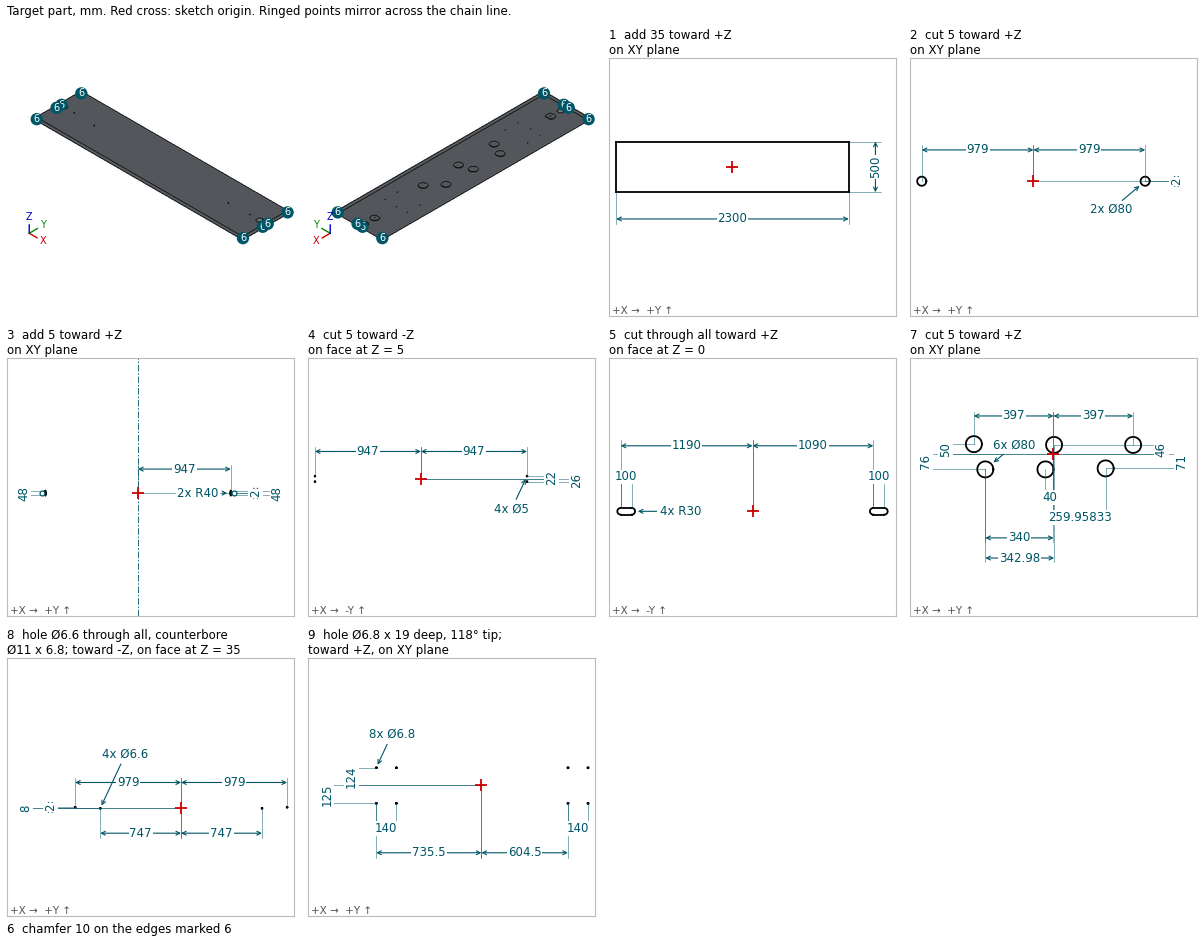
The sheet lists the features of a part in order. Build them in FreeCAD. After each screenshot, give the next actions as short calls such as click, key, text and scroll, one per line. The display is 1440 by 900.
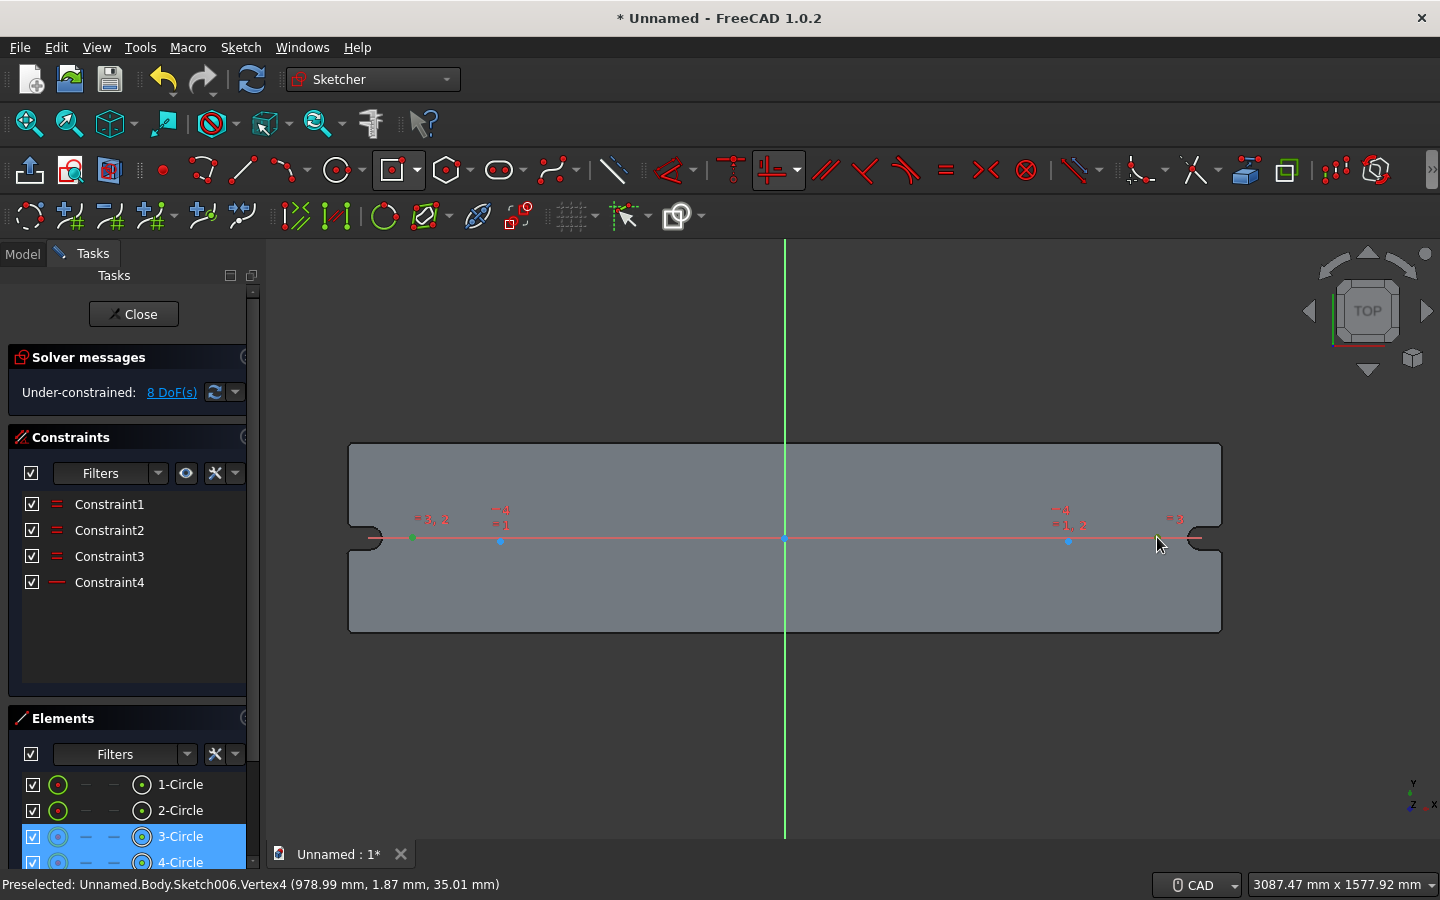
click(800, 170)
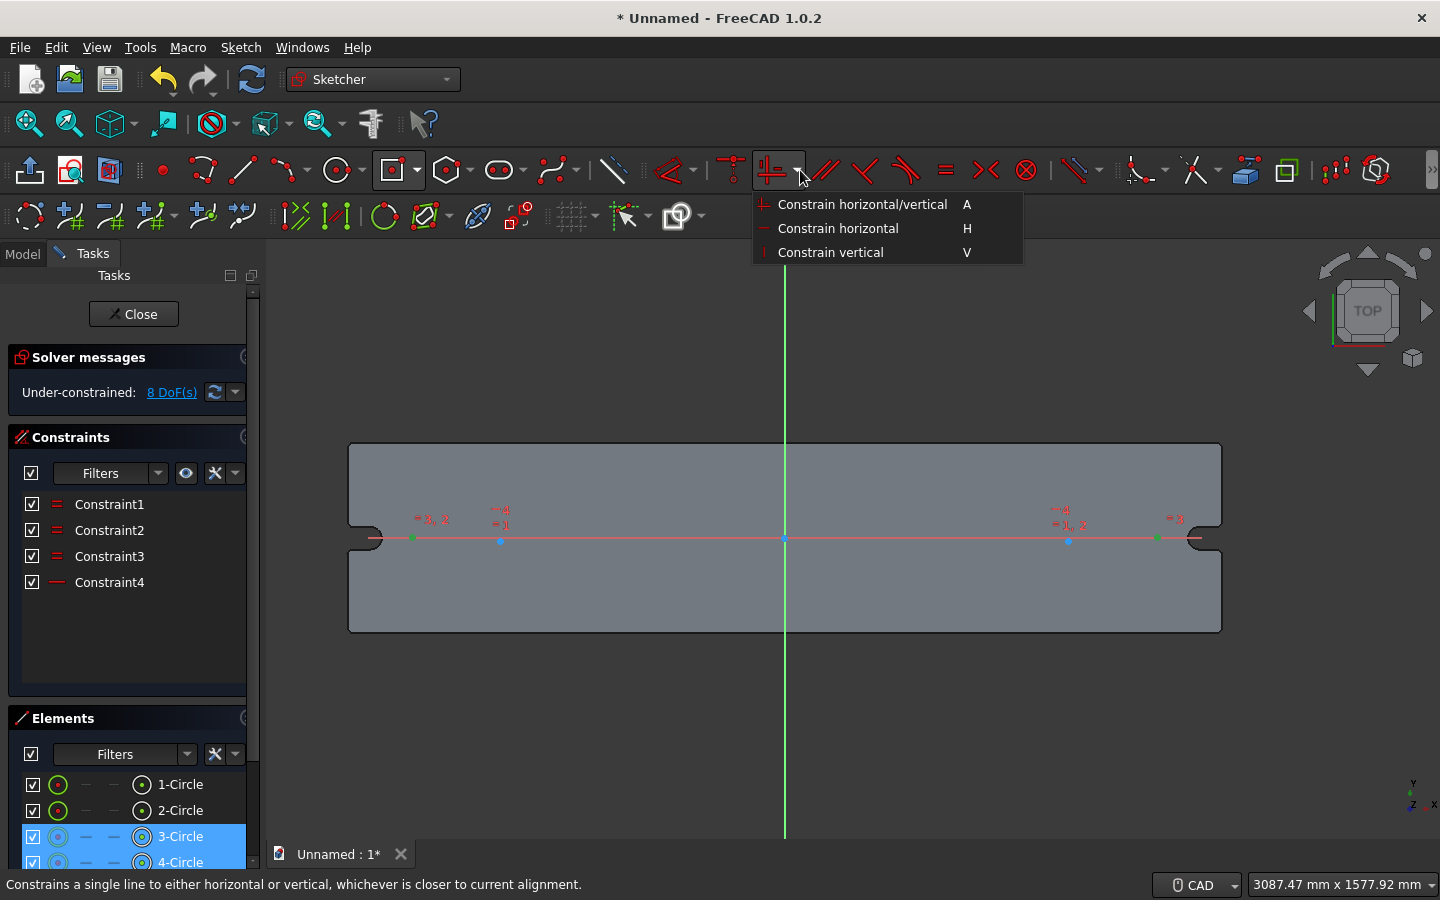
click(888, 228)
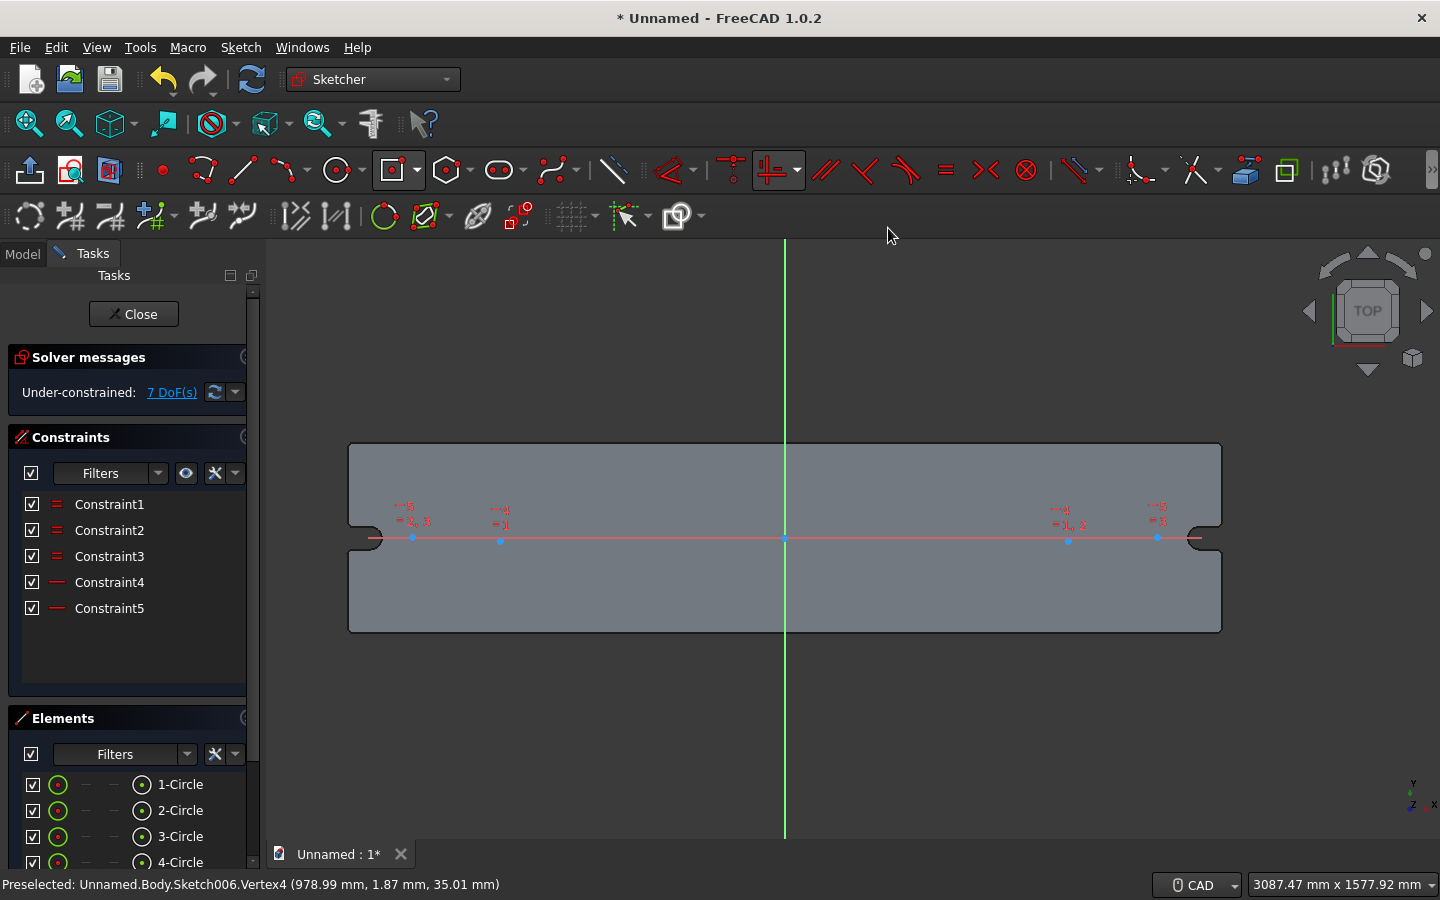
click(668, 170)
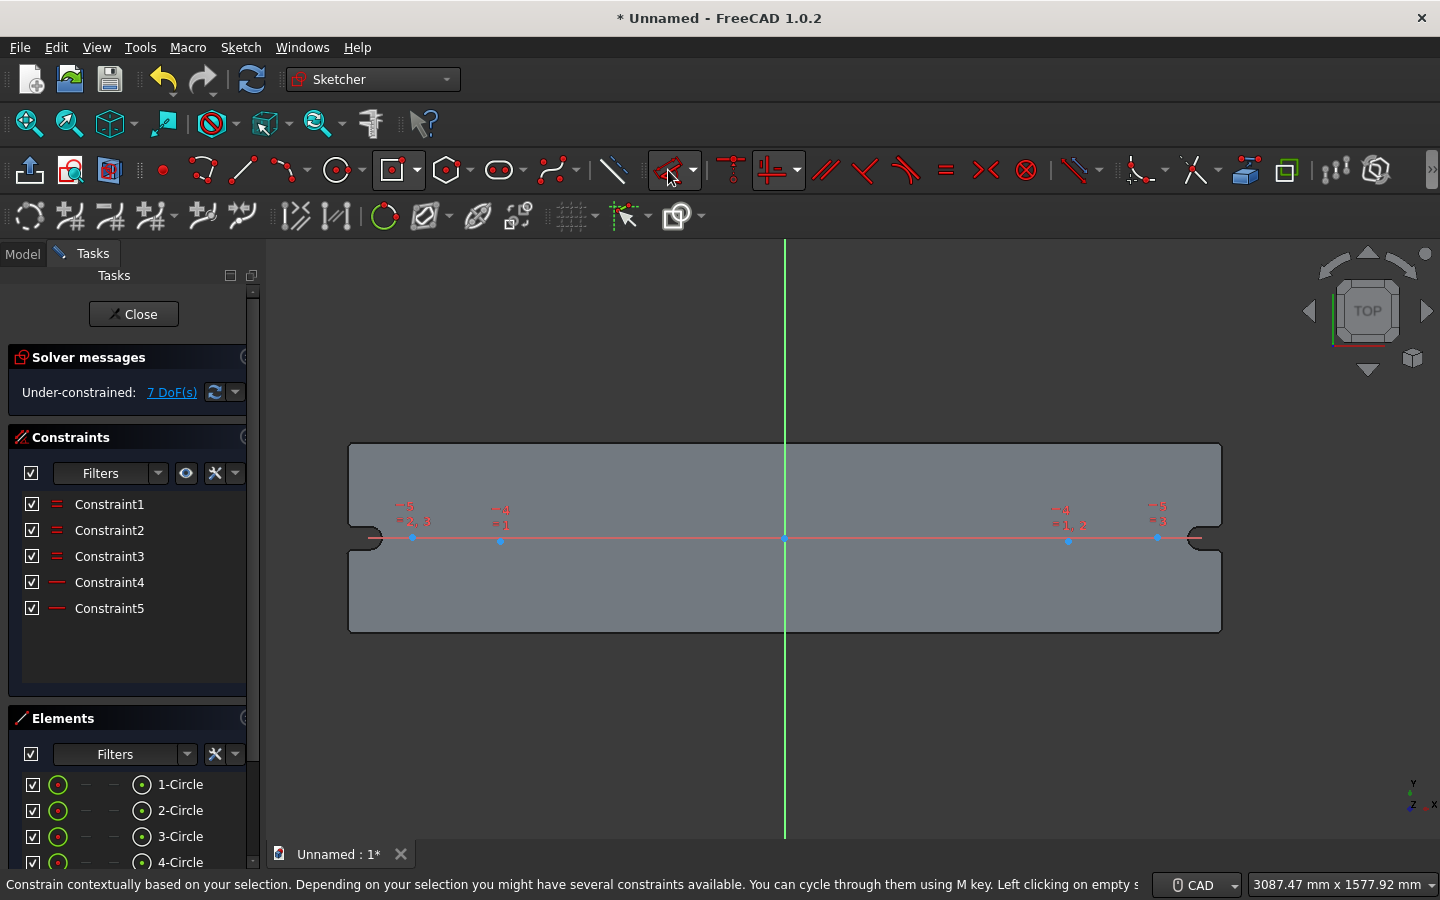
scroll(501, 540, up, 14)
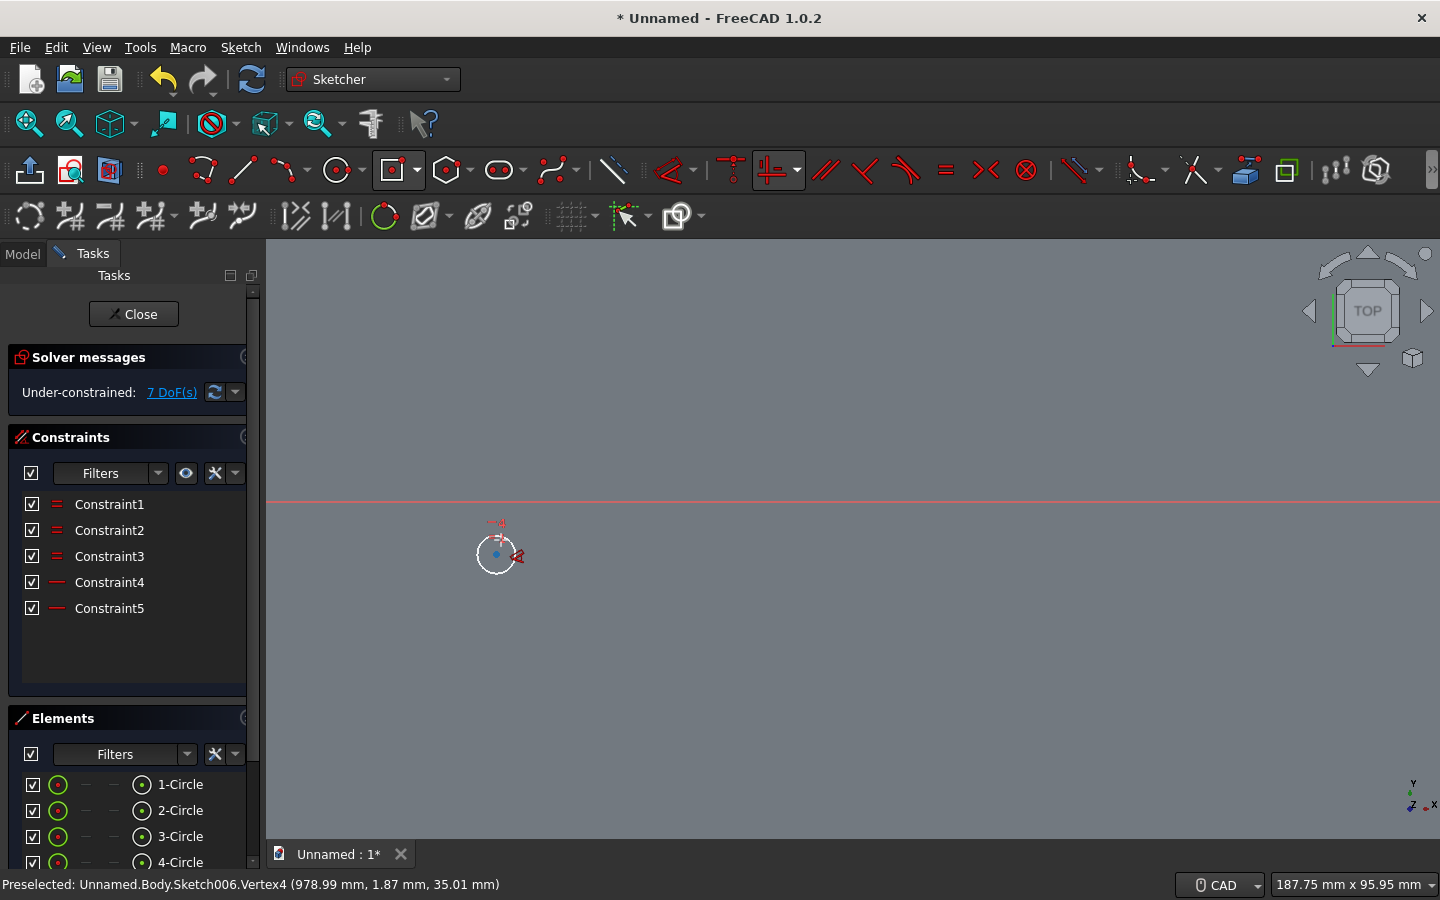
click(497, 536)
click(540, 529)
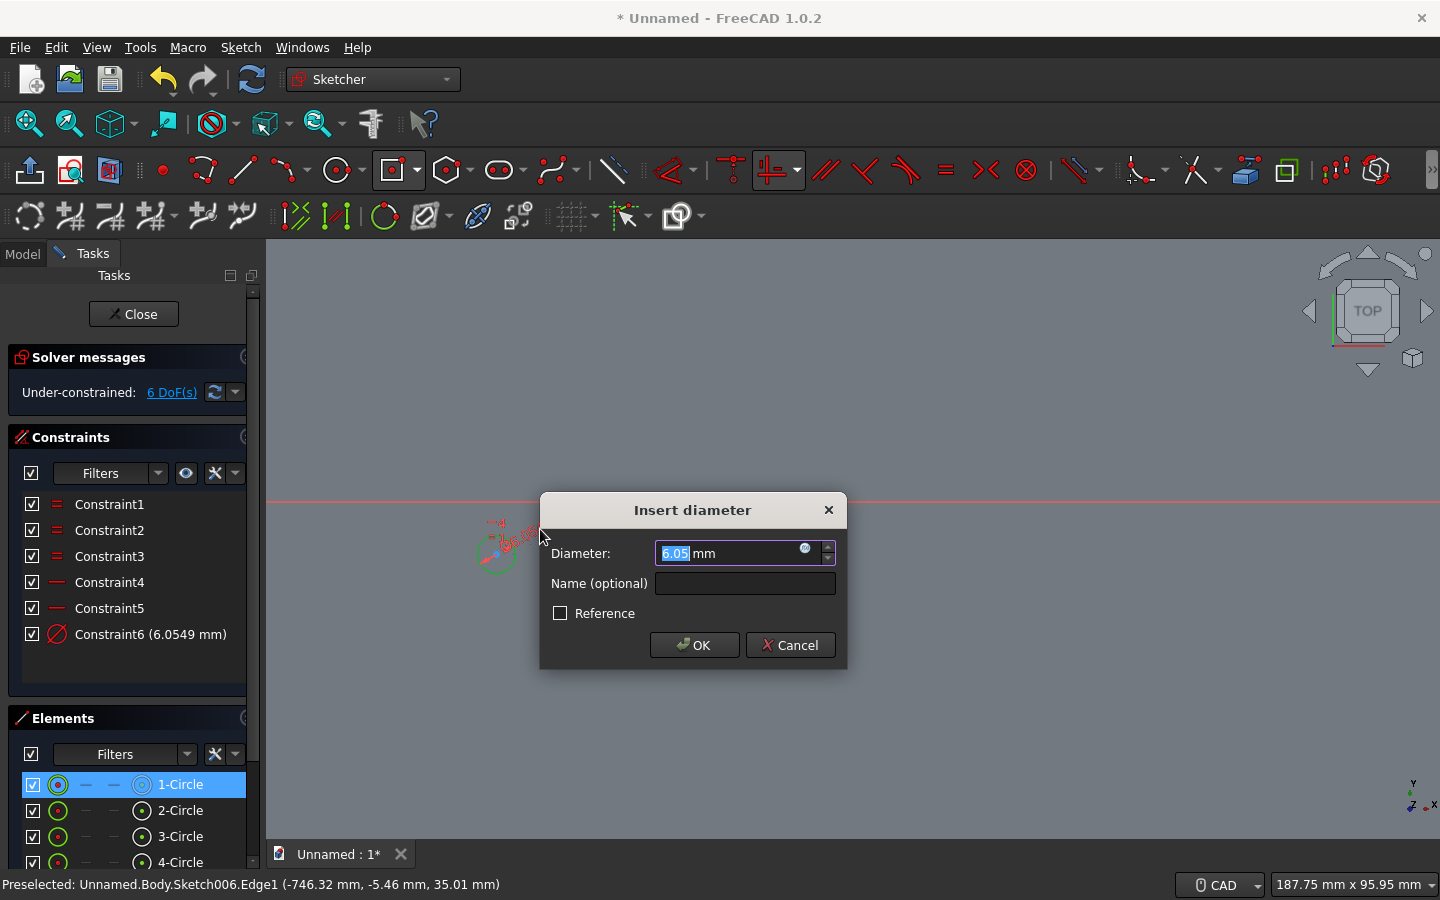
text(6.6)
key(Return)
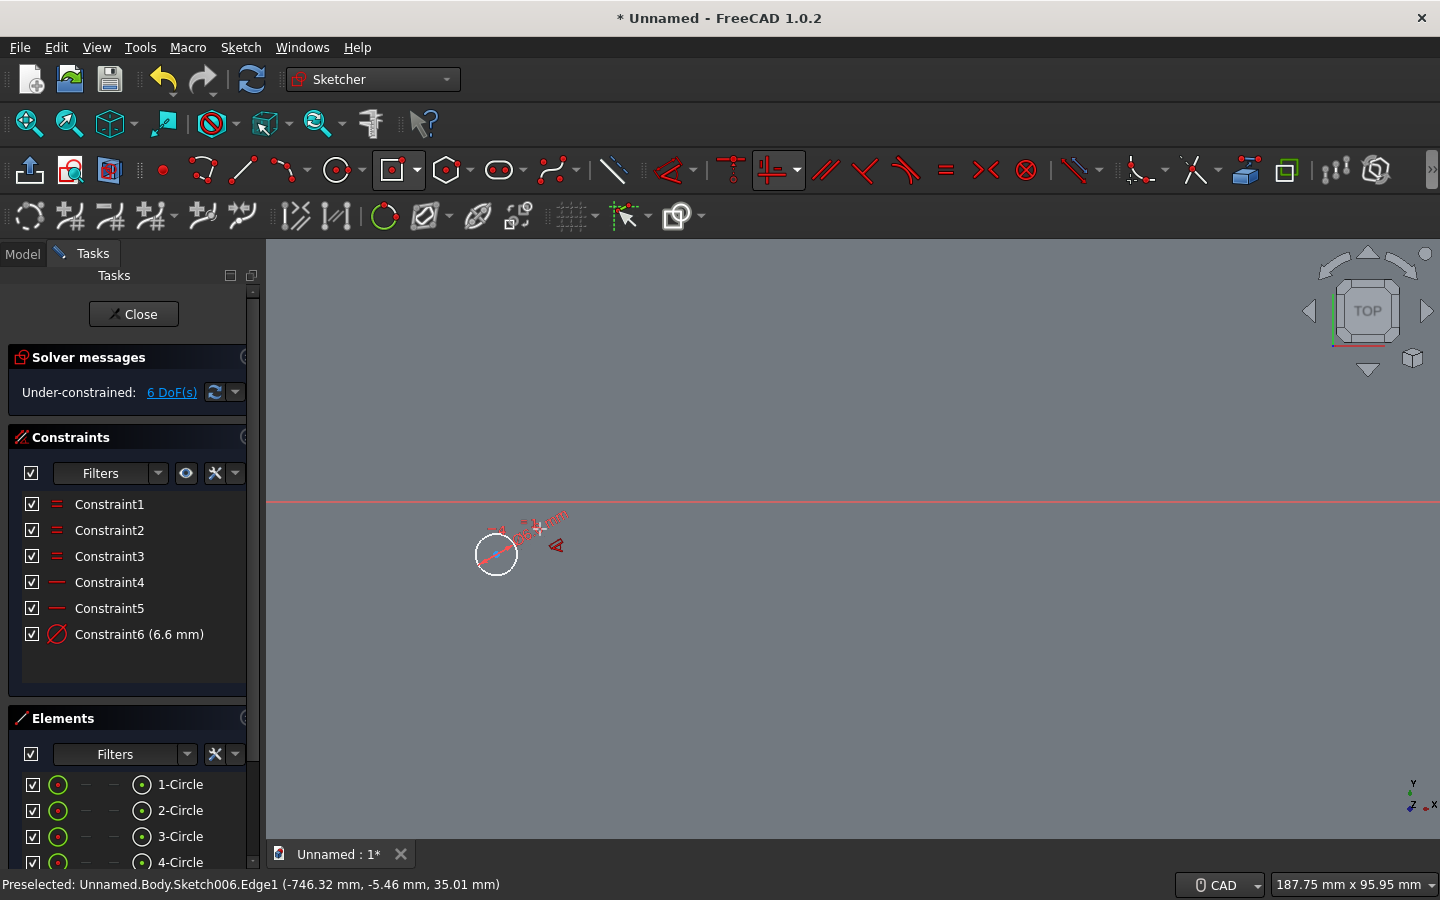
click(496, 555)
click(462, 528)